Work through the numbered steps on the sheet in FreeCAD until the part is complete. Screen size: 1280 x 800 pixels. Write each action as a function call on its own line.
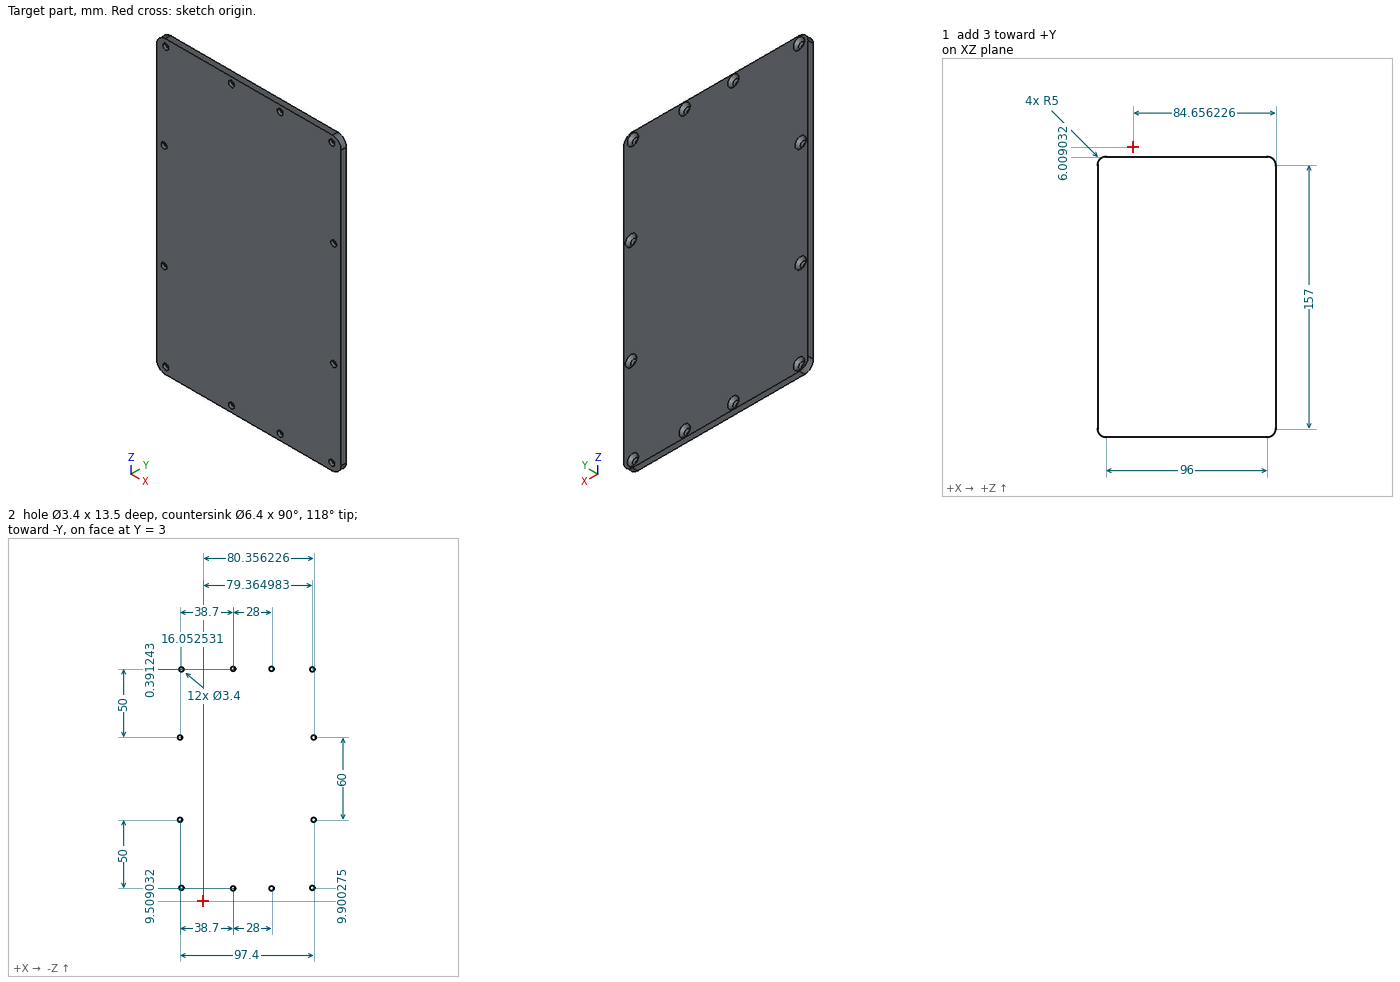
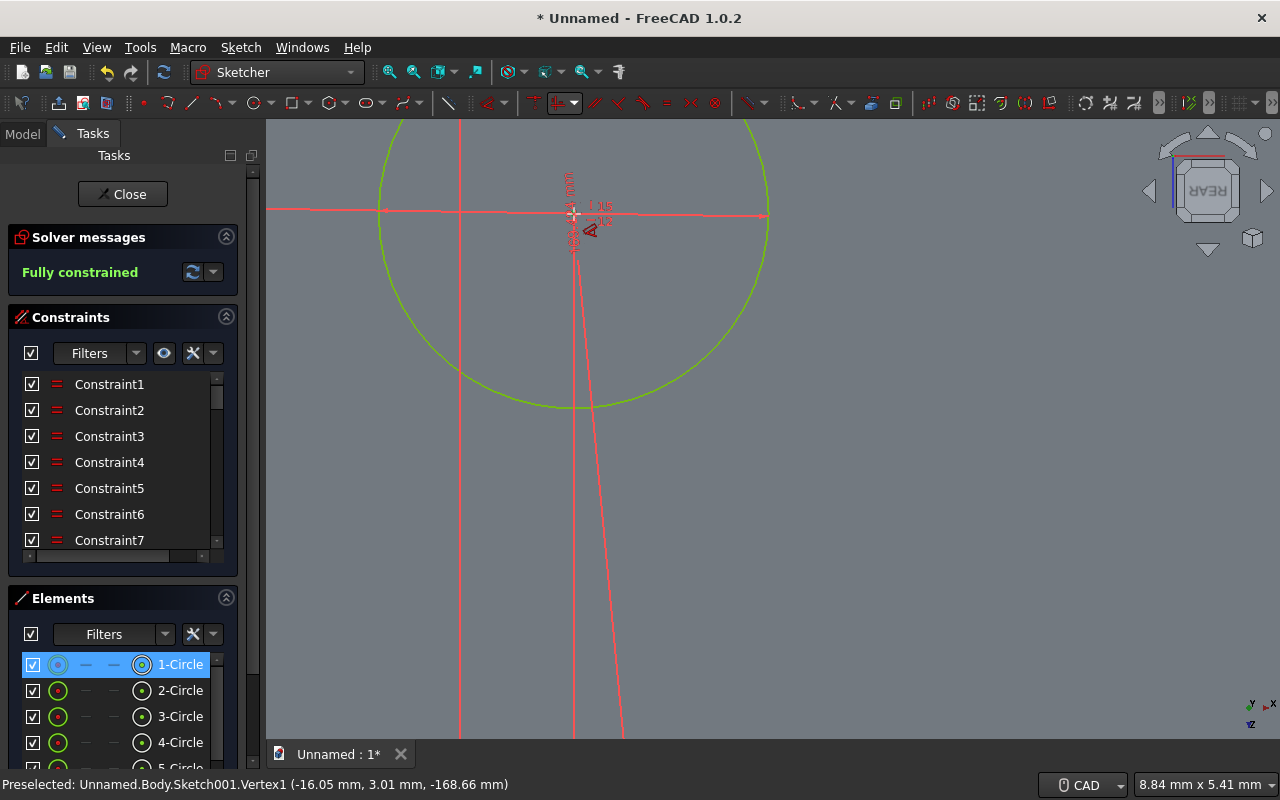
scroll(704, 429, down, 15)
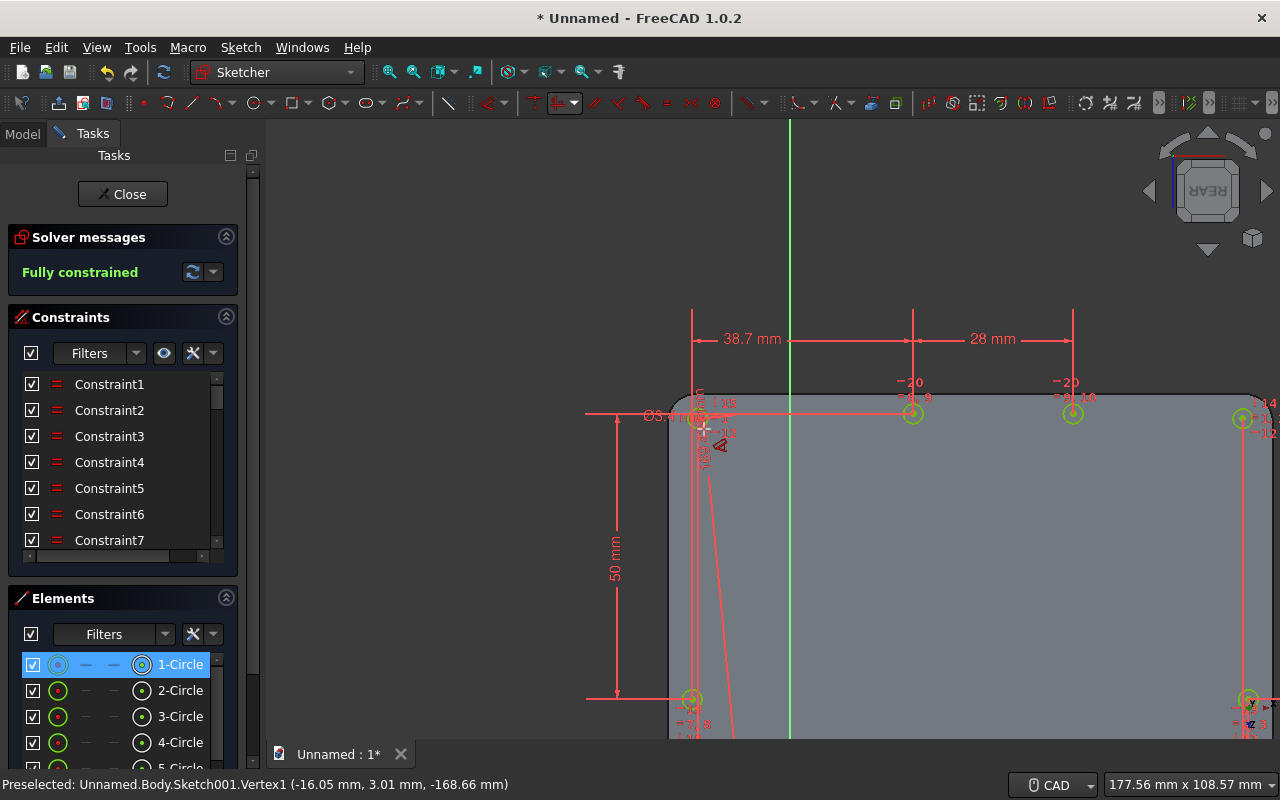
scroll(550, 159, down, 5)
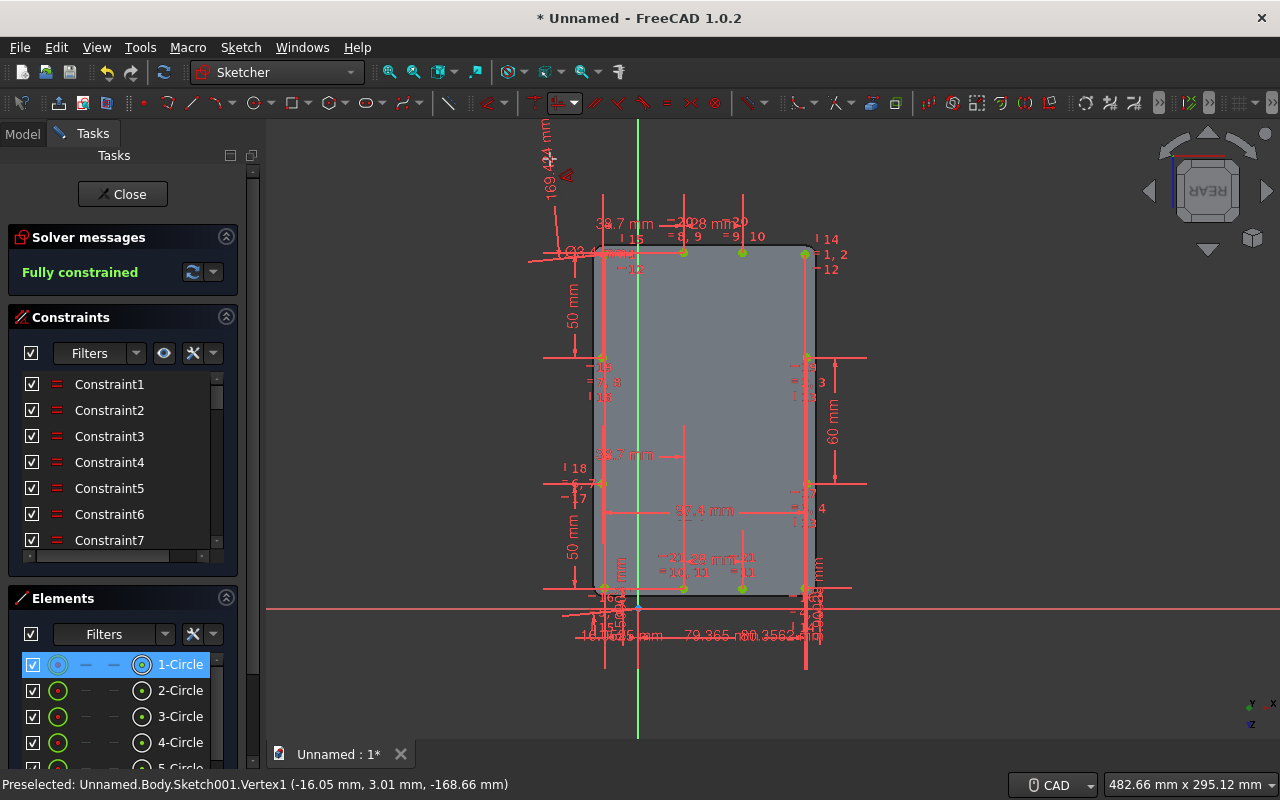
scroll(684, 253, up, 20)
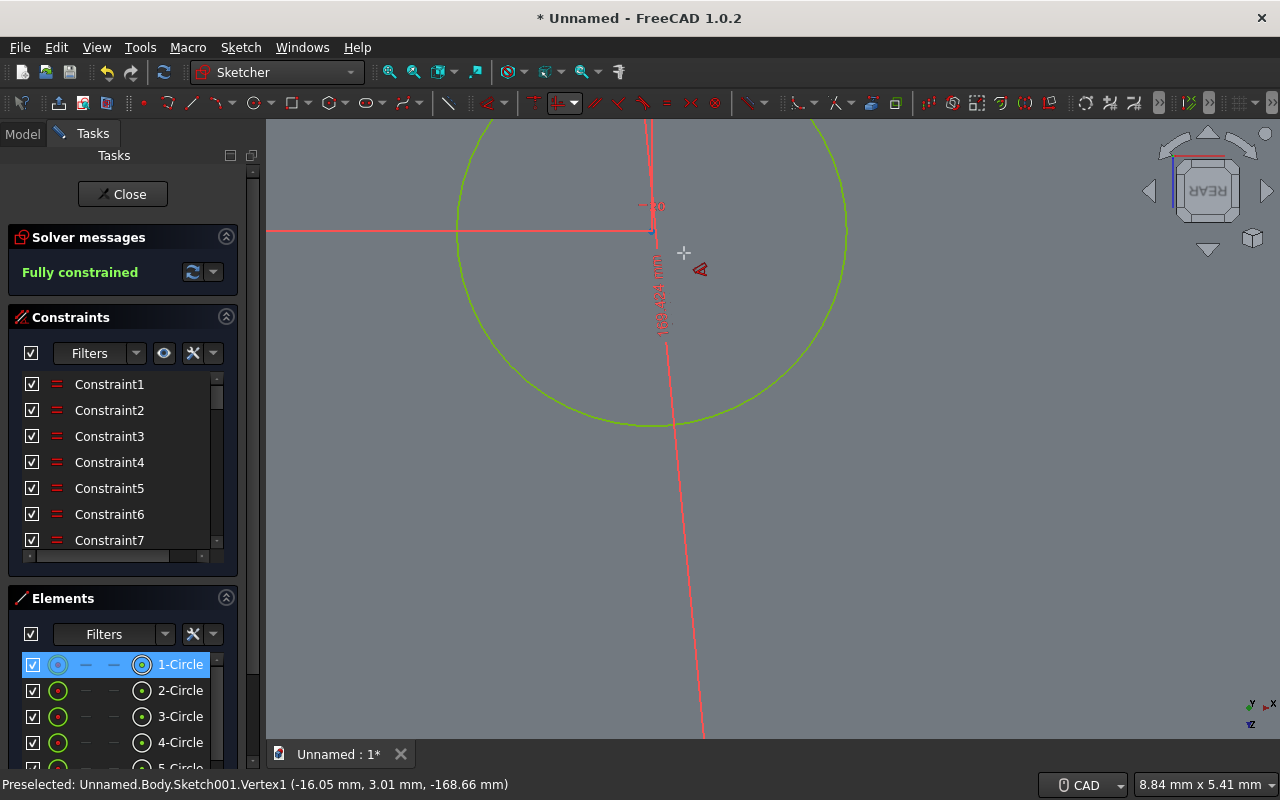
click(652, 231)
click(686, 280)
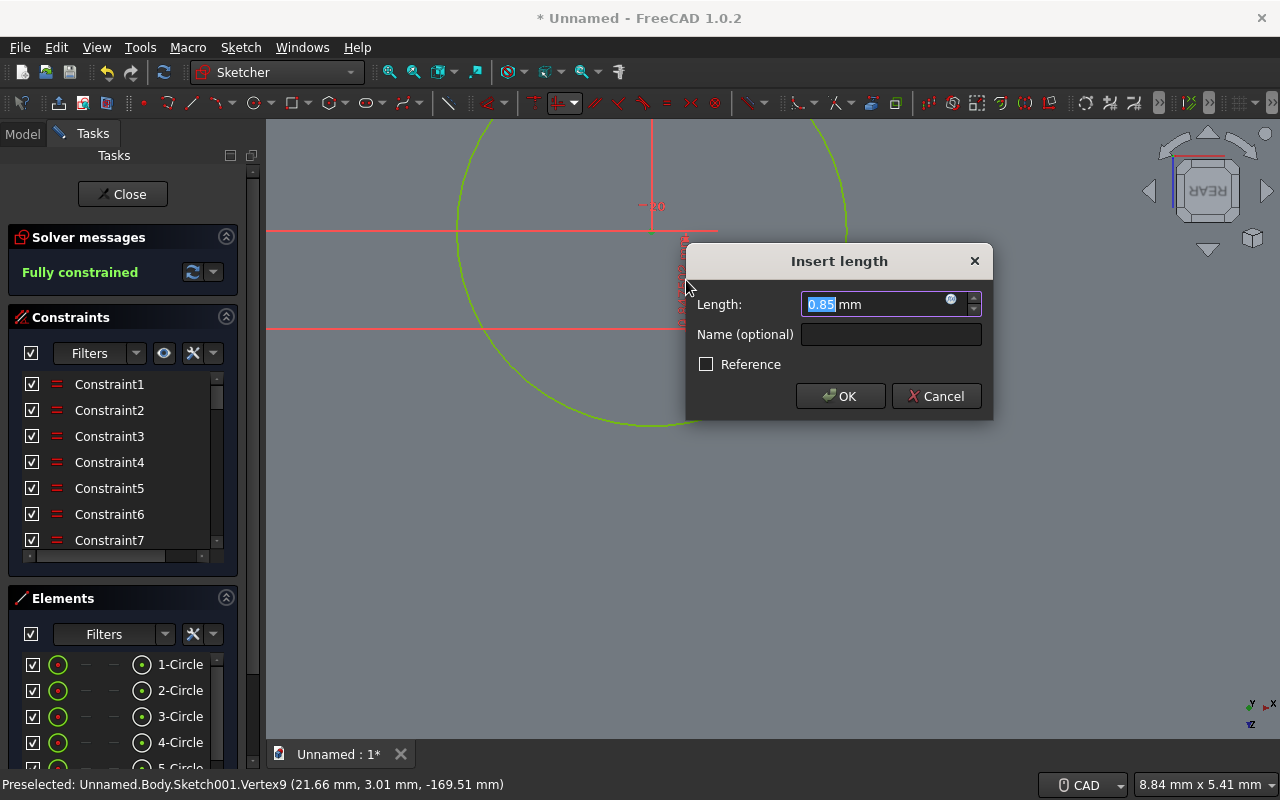
text(0.391243)
key(Return)
key(Escape)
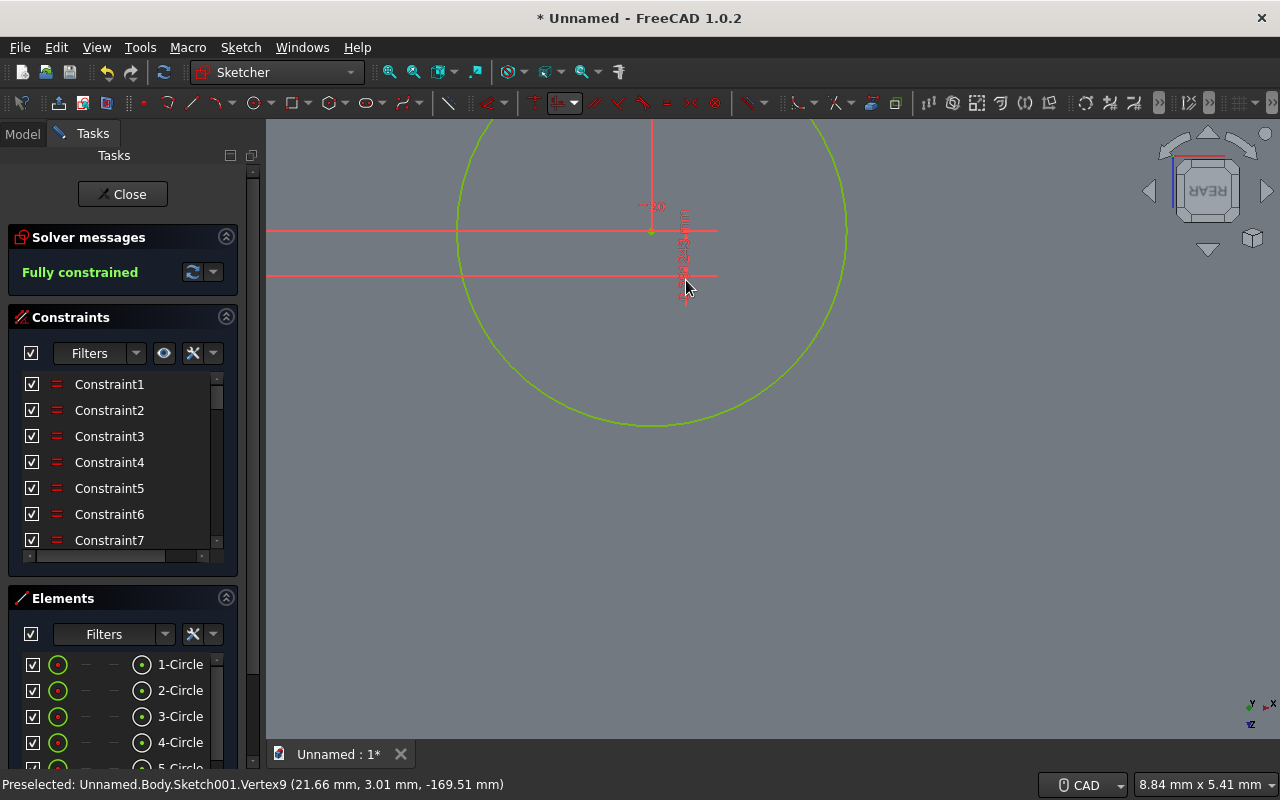
click(123, 194)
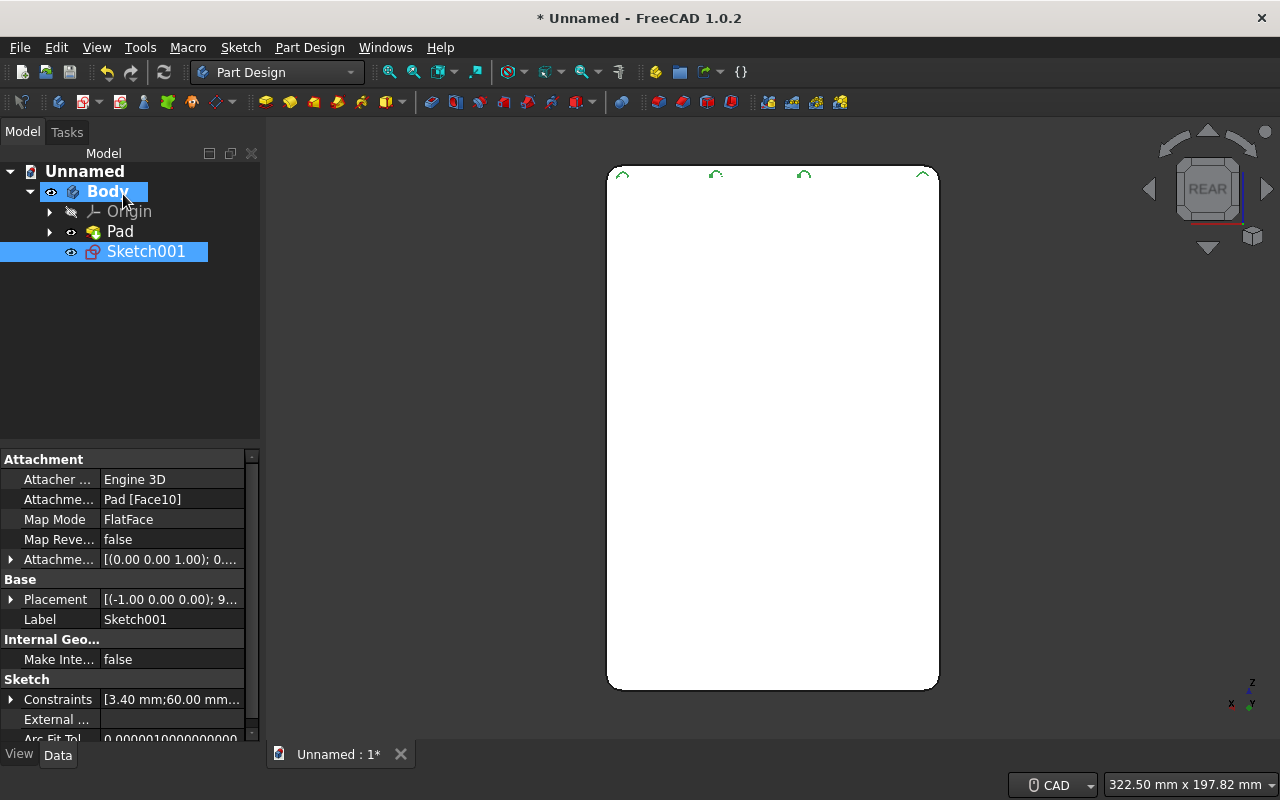
click(456, 102)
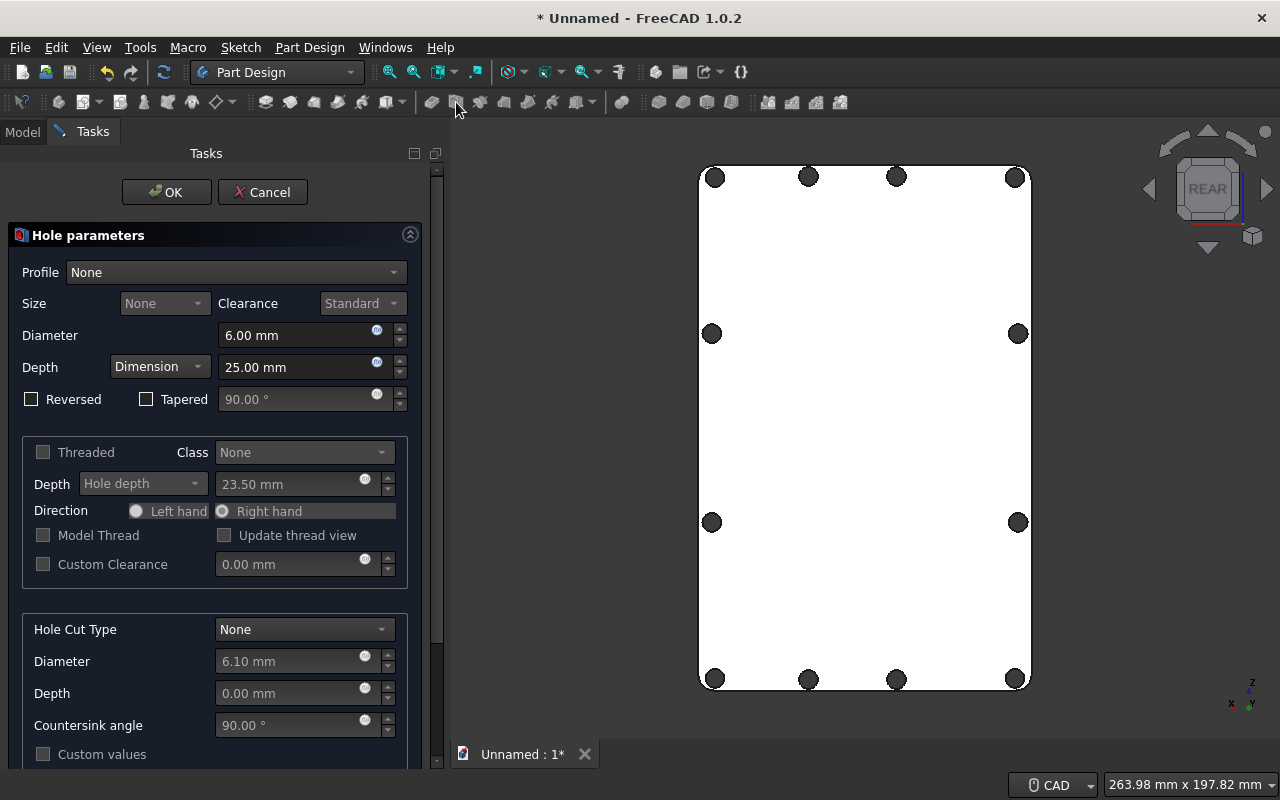
triple_click(305, 335)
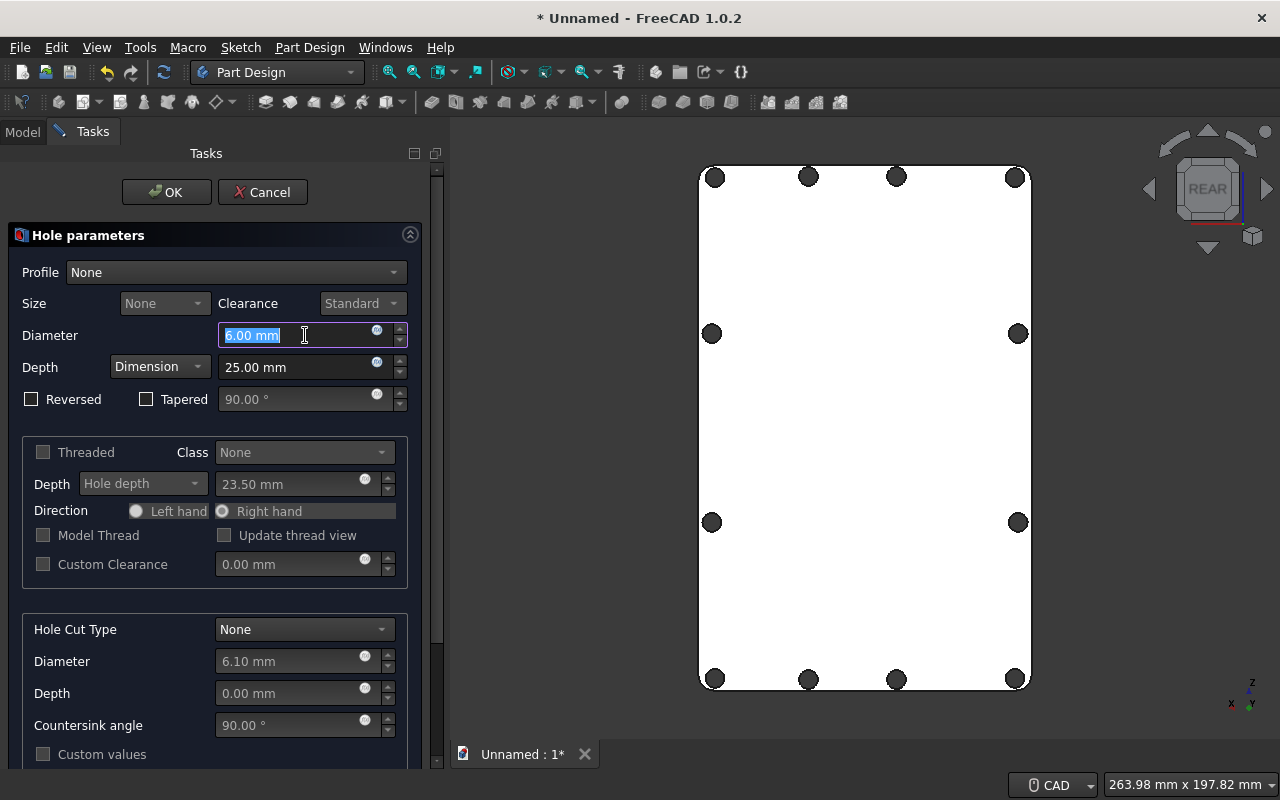
text(3.4)
key(Tab)